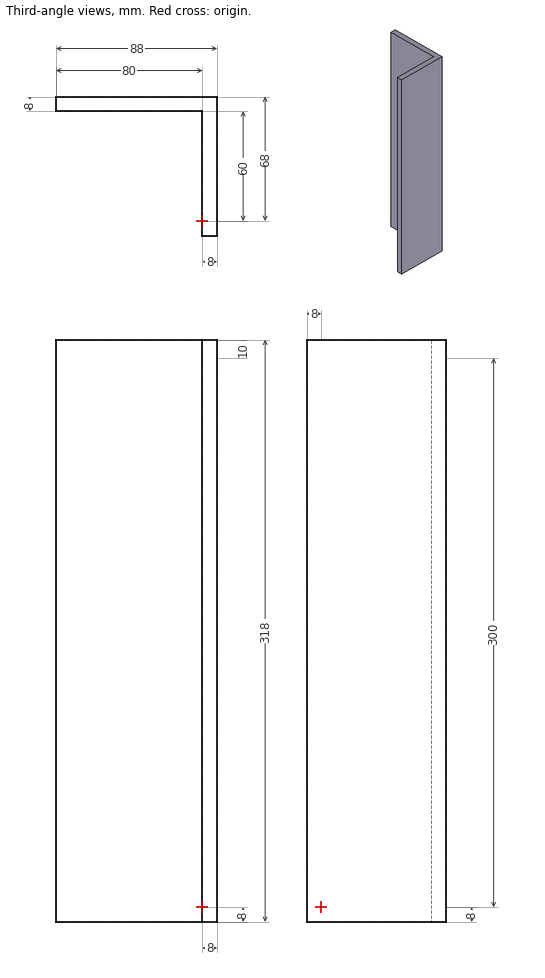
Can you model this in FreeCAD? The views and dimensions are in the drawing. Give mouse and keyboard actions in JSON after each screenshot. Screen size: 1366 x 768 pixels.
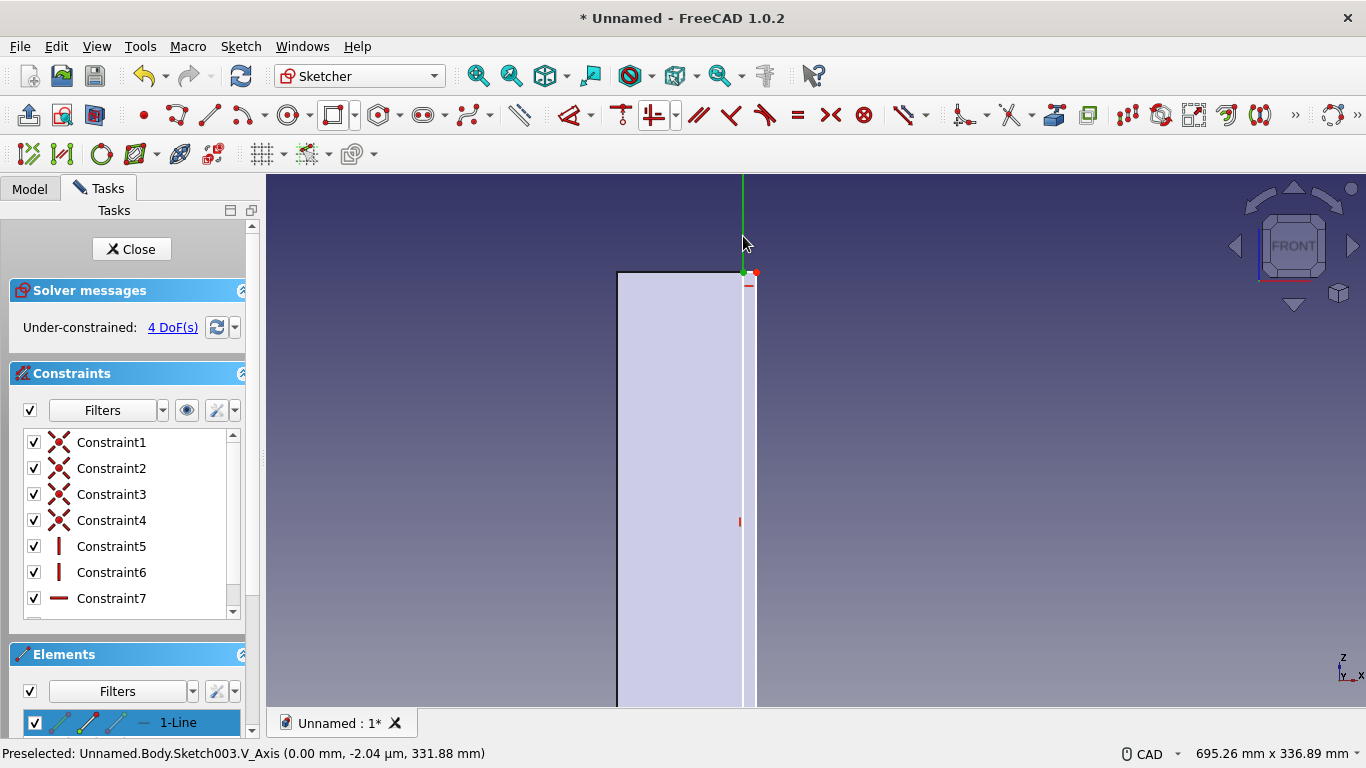
{"action": "left_click", "coordinate": [621, 116]}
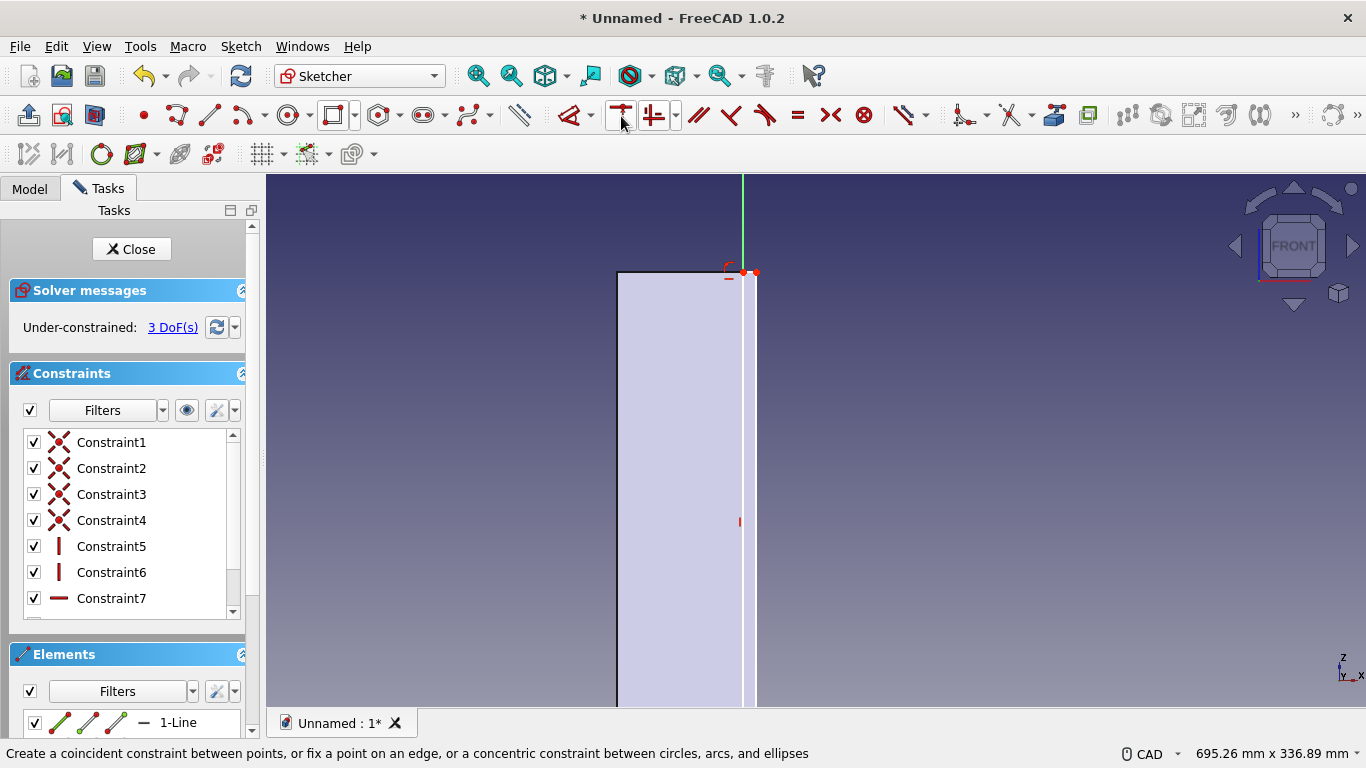
{"action": "key", "text": "d"}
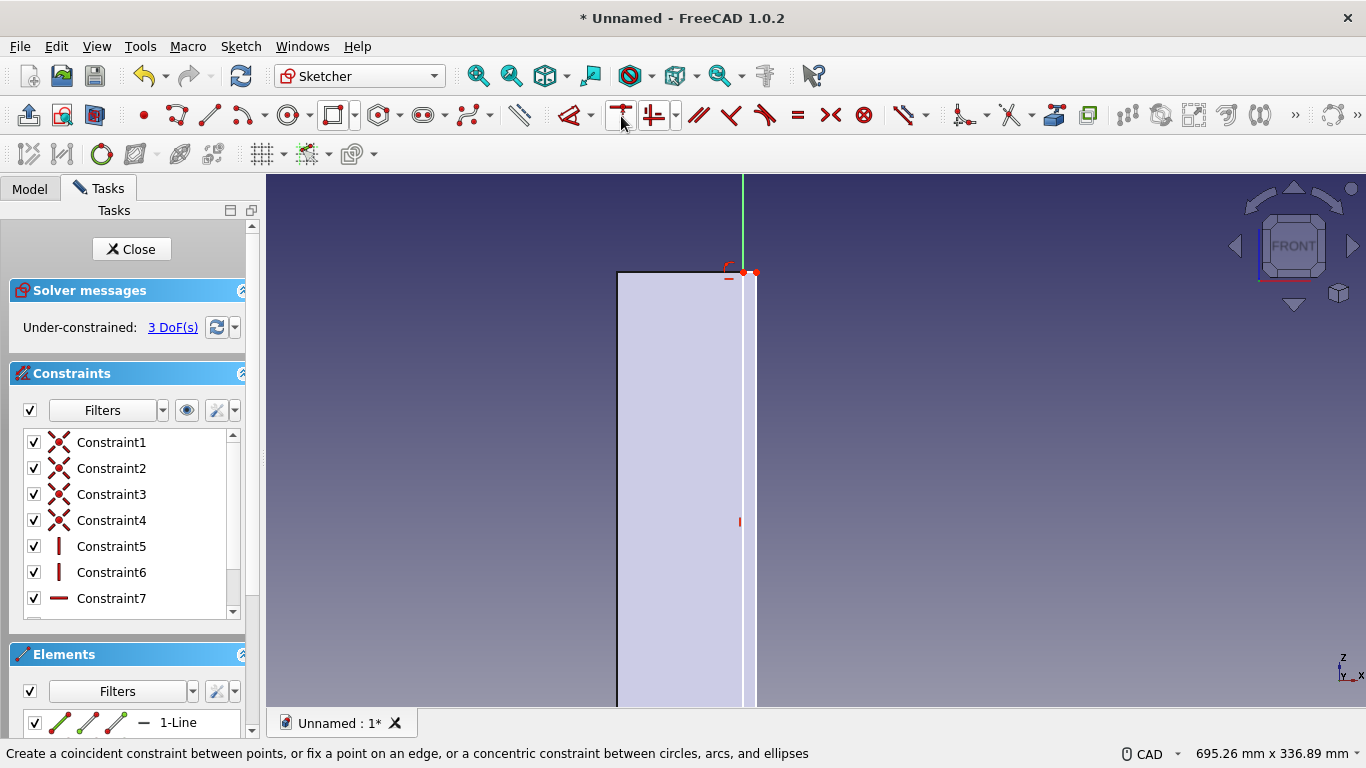
{"action": "scroll", "coordinate": [743, 272], "scroll_direction": "down", "scroll_amount": 2}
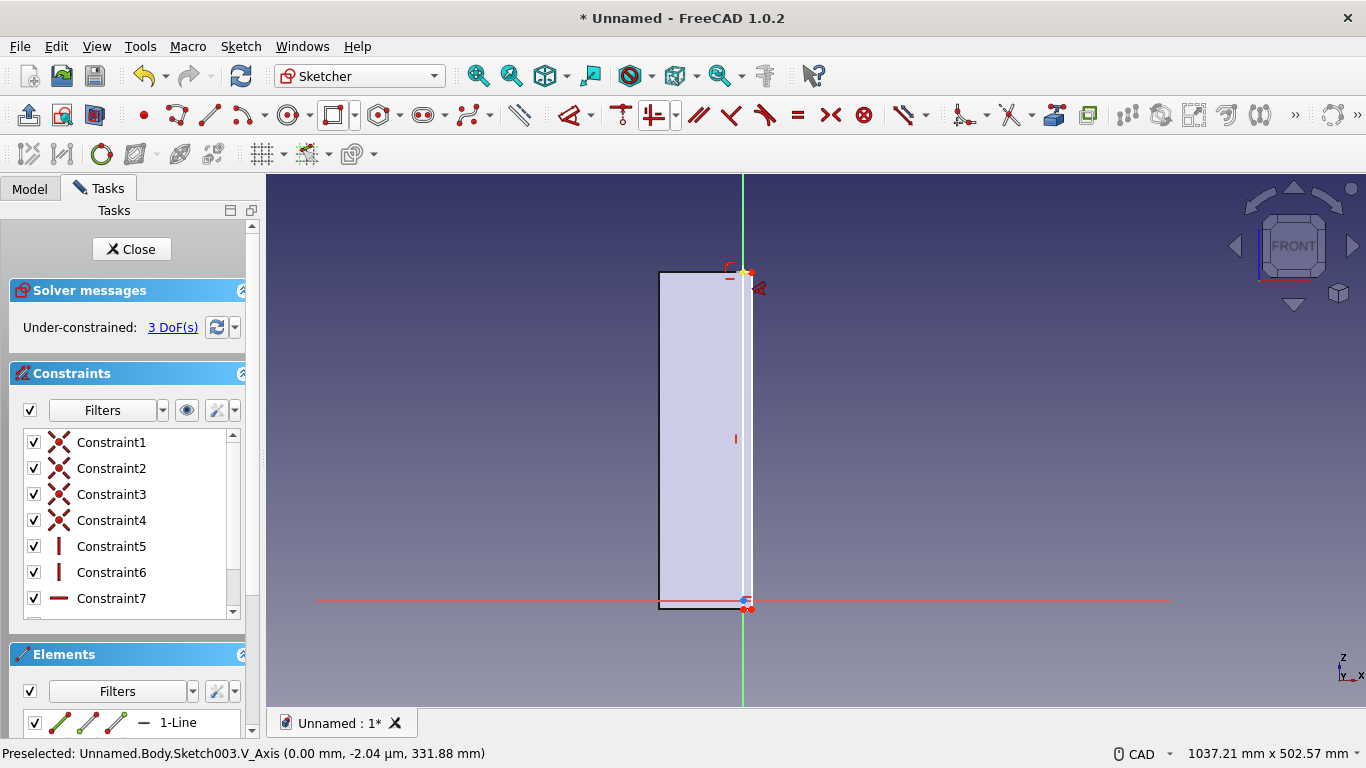
{"action": "scroll", "coordinate": [748, 610], "scroll_direction": "up", "scroll_amount": 8}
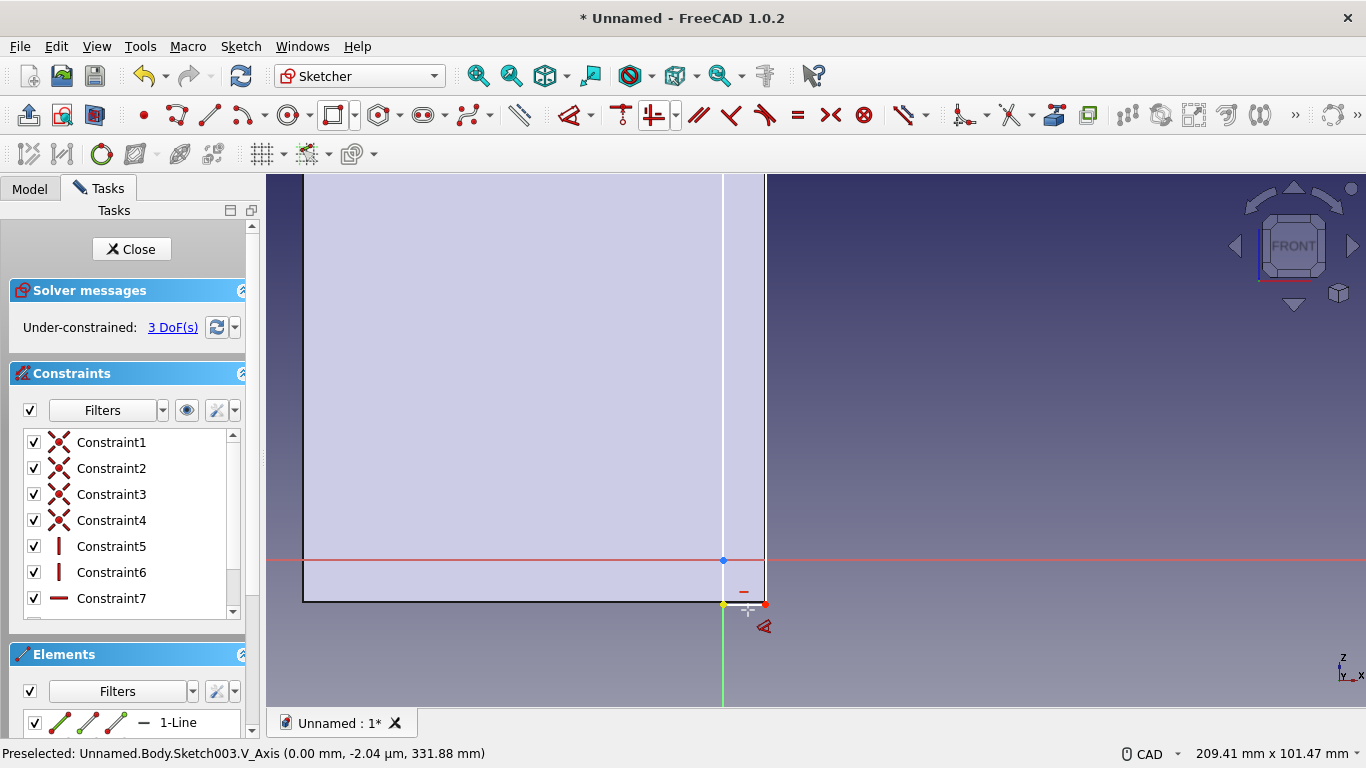
{"action": "left_click", "coordinate": [744, 605]}
{"action": "left_click", "coordinate": [744, 639]}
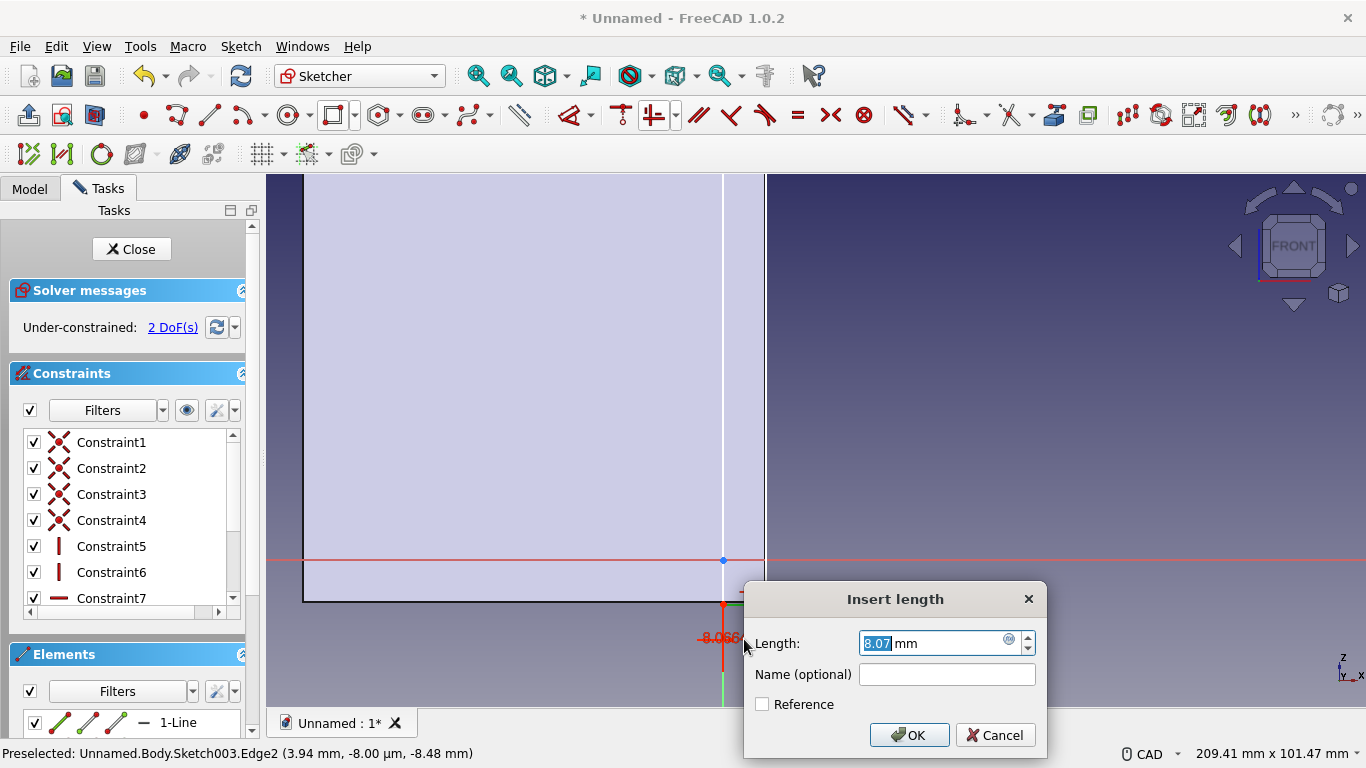
{"action": "type", "text": "8"}
{"action": "key", "text": "Return"}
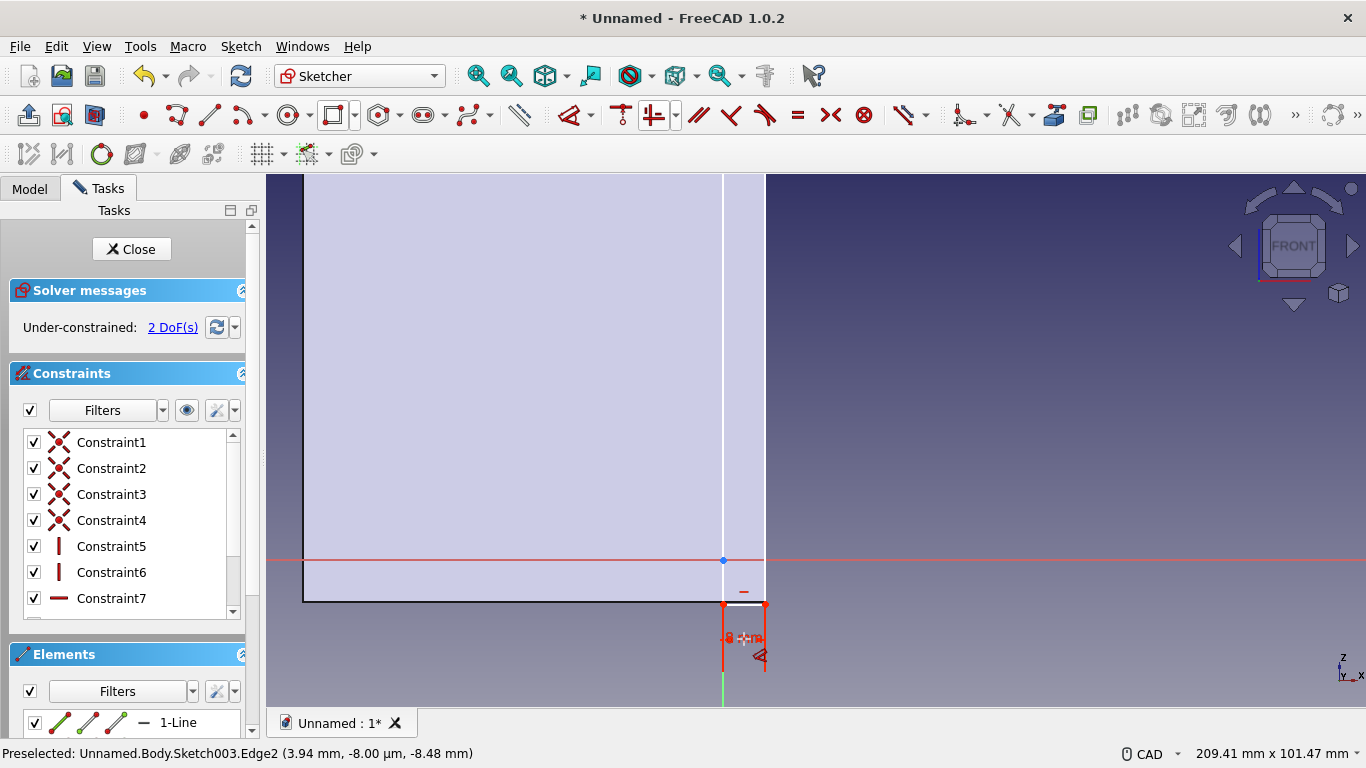
{"action": "left_click", "coordinate": [723, 605]}
{"action": "left_click", "coordinate": [689, 582]}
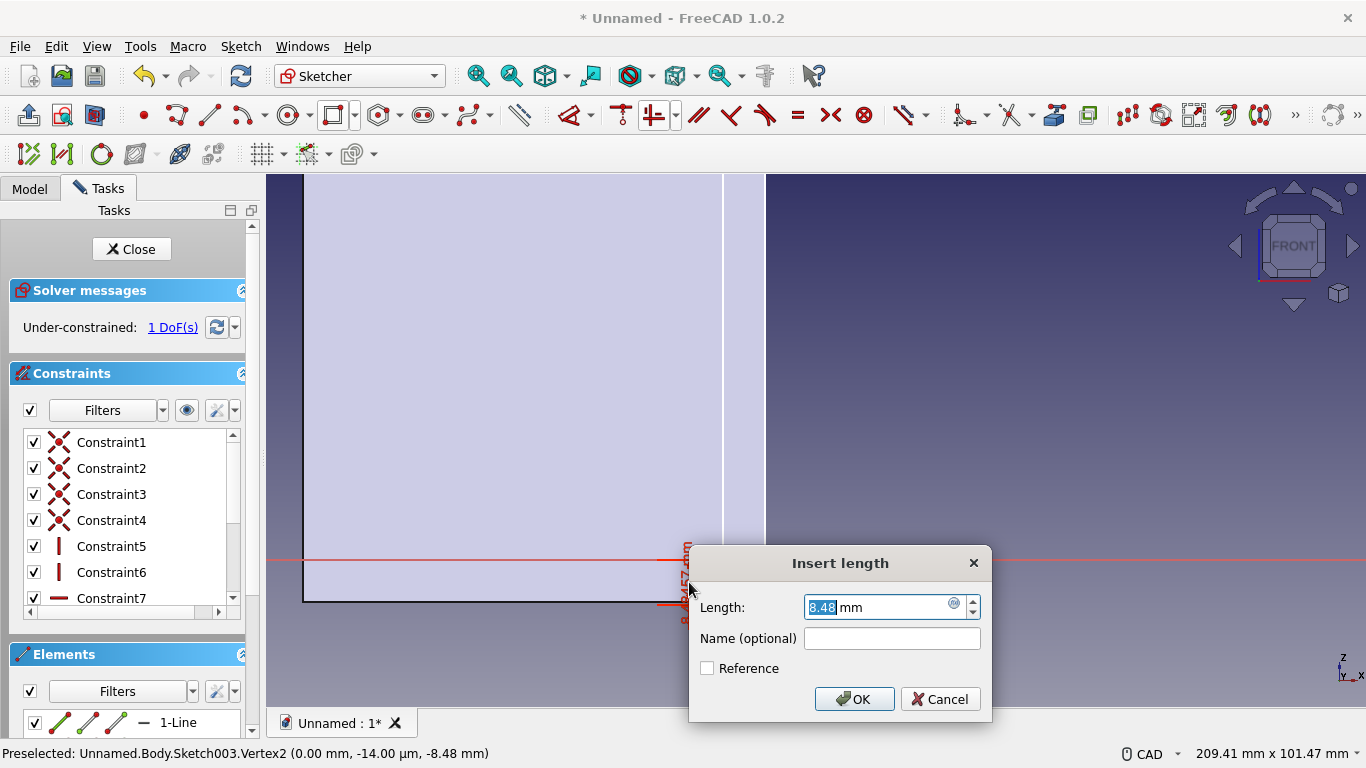
{"action": "type", "text": "8"}
{"action": "key", "text": "Return"}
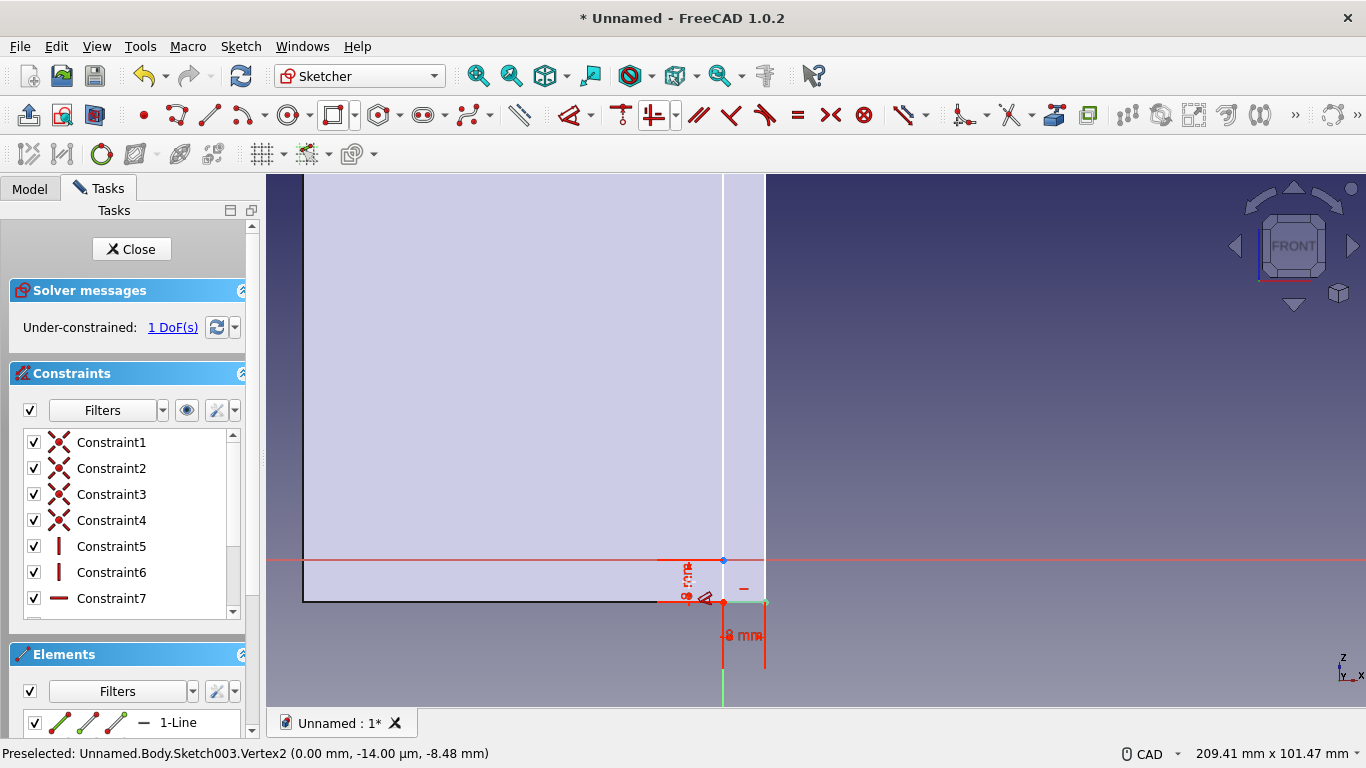
{"action": "scroll", "coordinate": [748, 611], "scroll_direction": "down", "scroll_amount": 8}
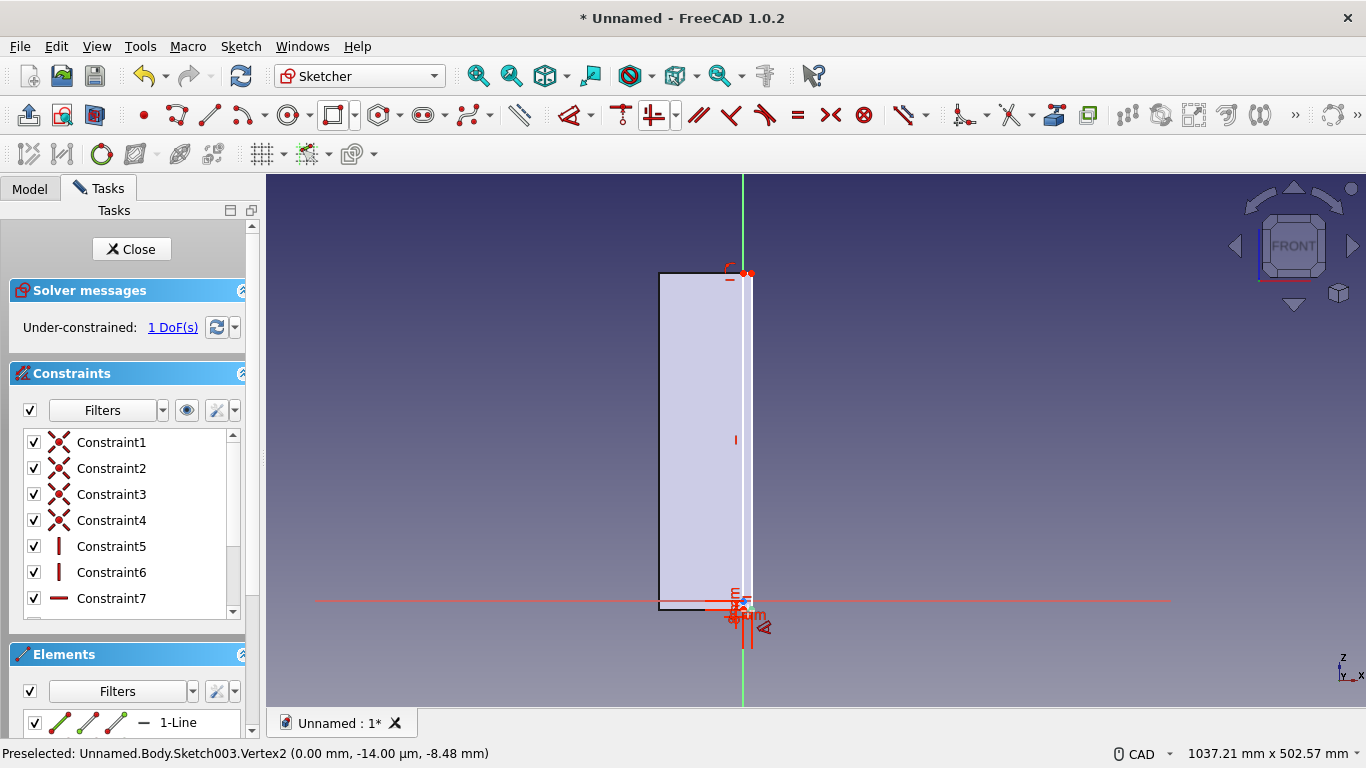
{"action": "scroll", "coordinate": [743, 542], "scroll_direction": "up", "scroll_amount": 3}